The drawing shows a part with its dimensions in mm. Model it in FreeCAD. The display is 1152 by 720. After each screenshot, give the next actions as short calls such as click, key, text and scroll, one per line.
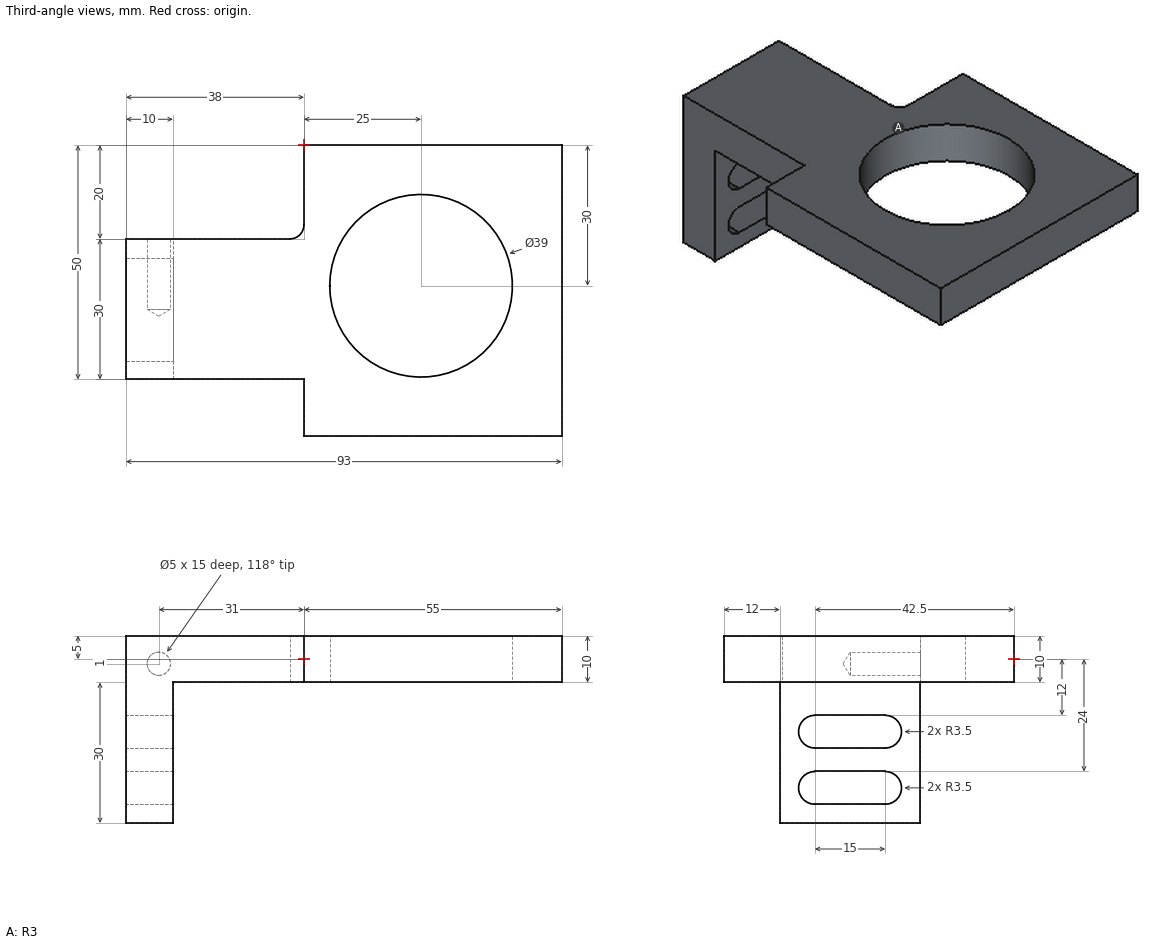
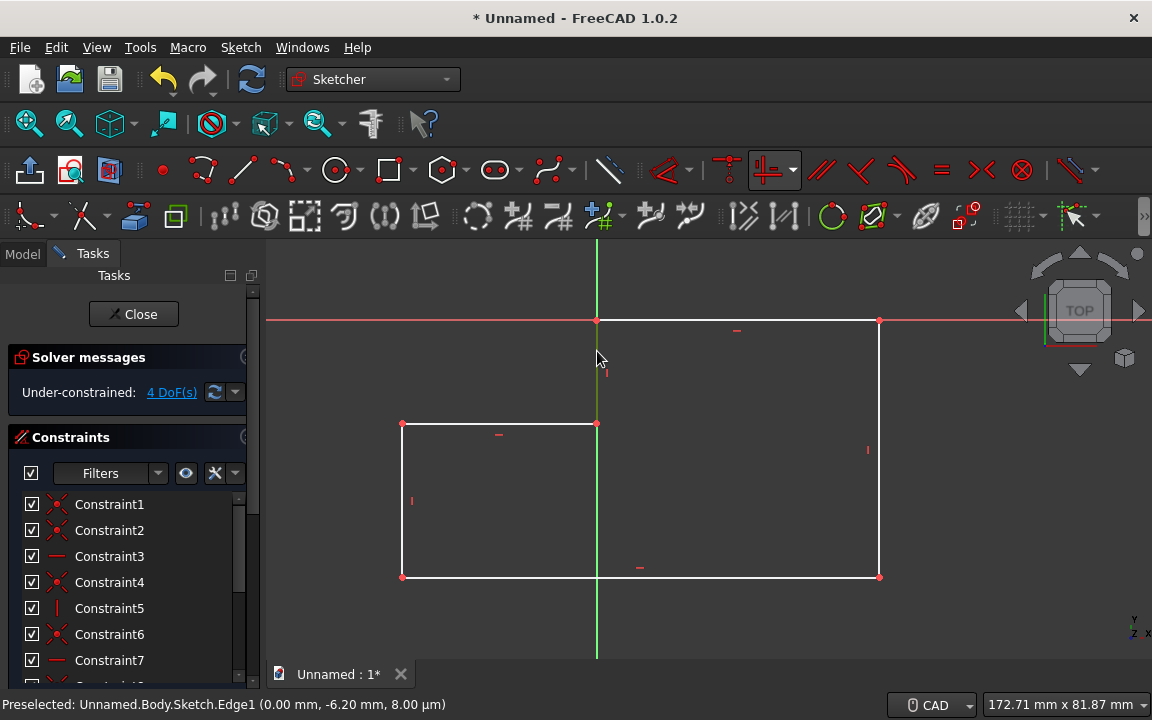
key(i)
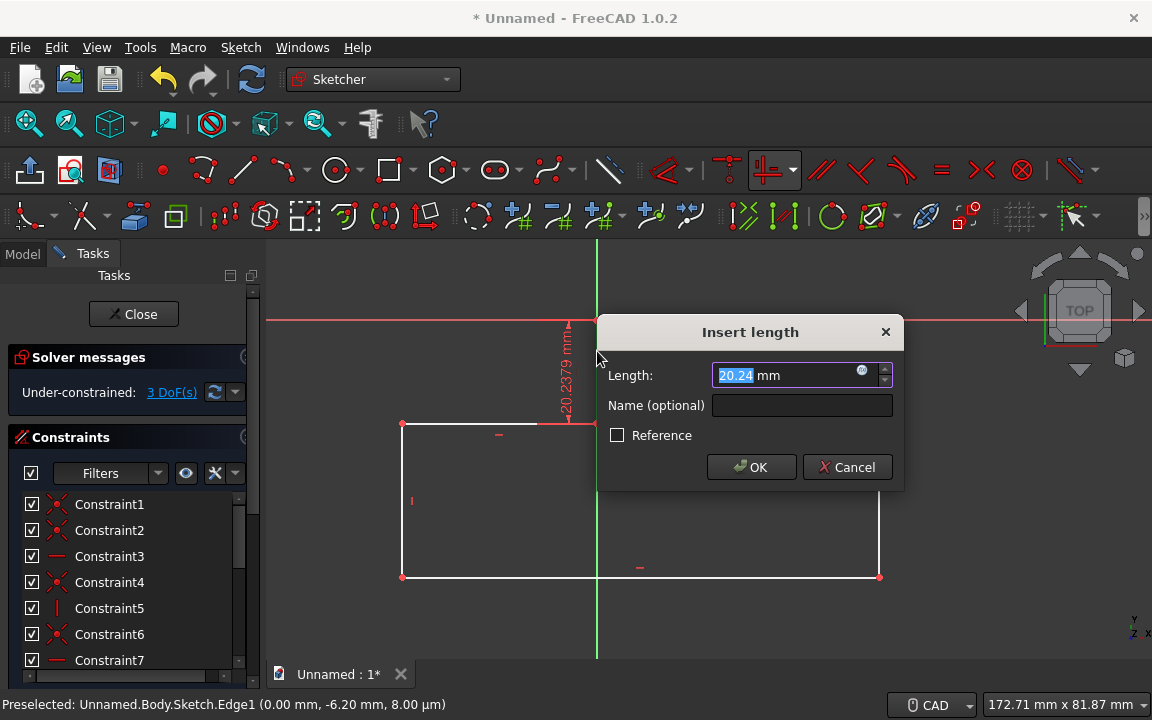
text(20)
key(Return)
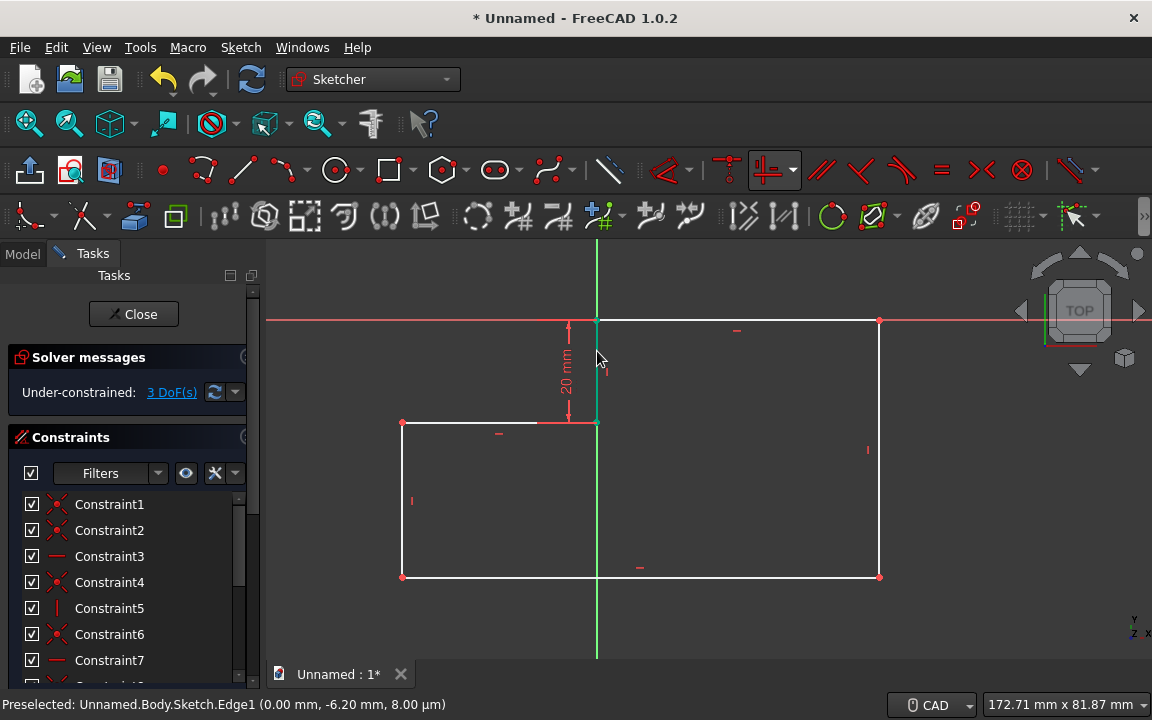
click(538, 423)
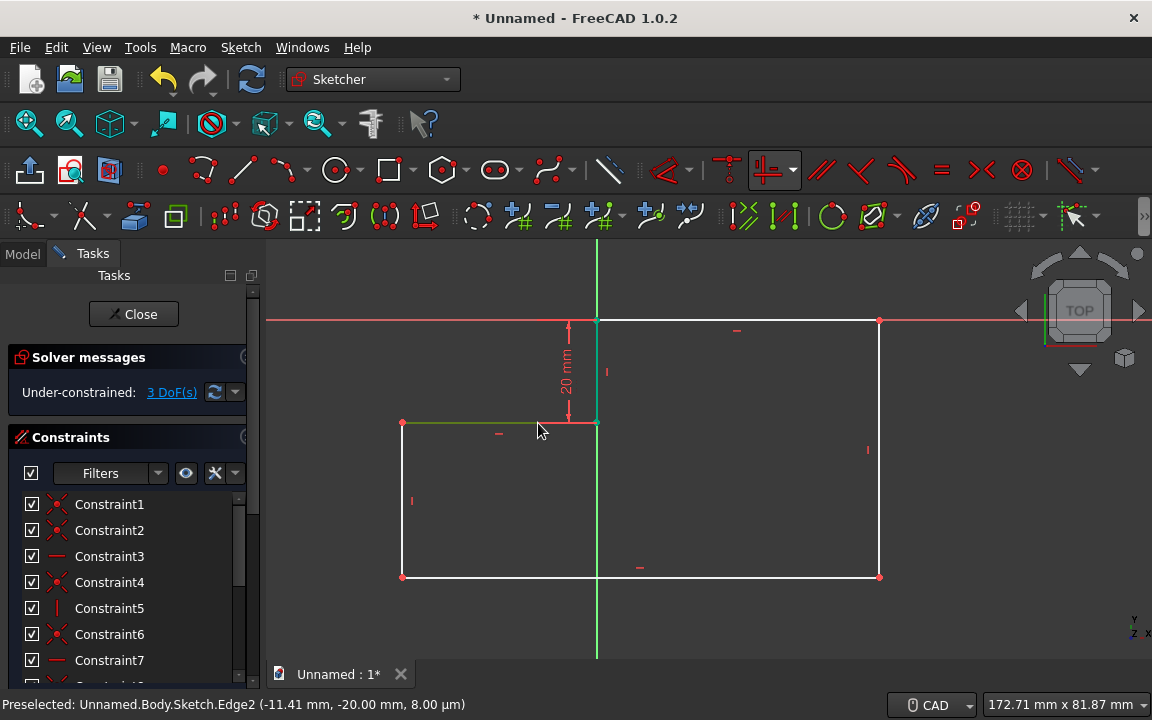
click(692, 170)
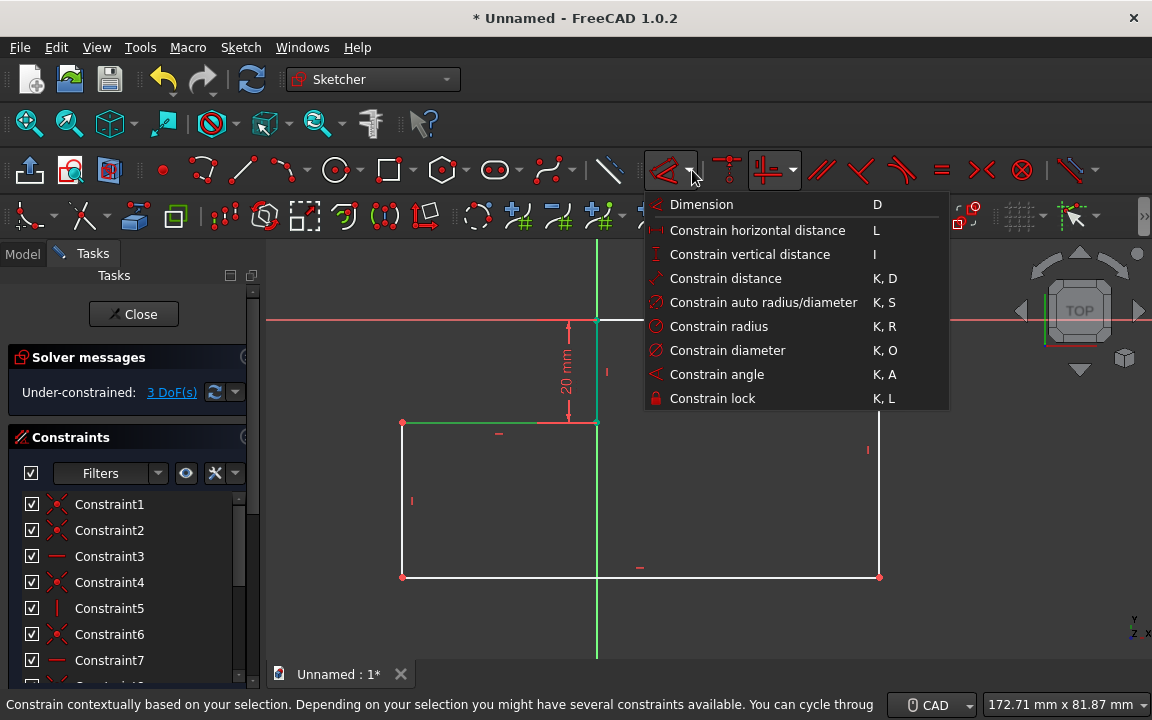
click(797, 230)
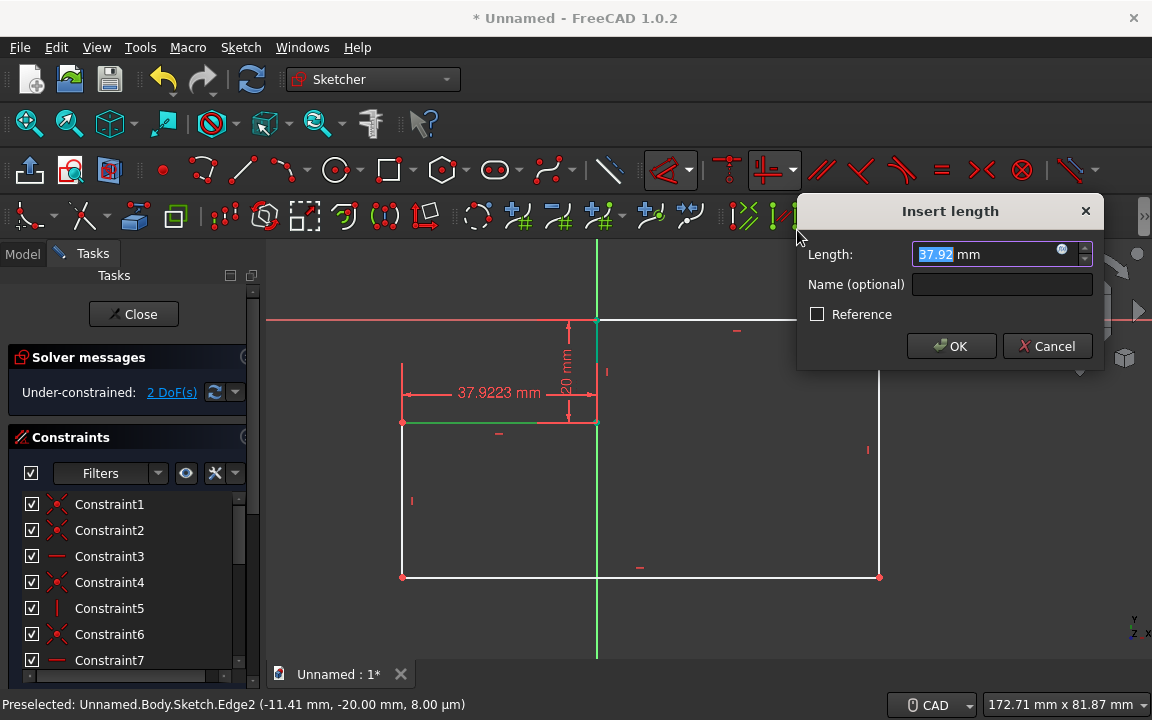
text(38)
key(Return)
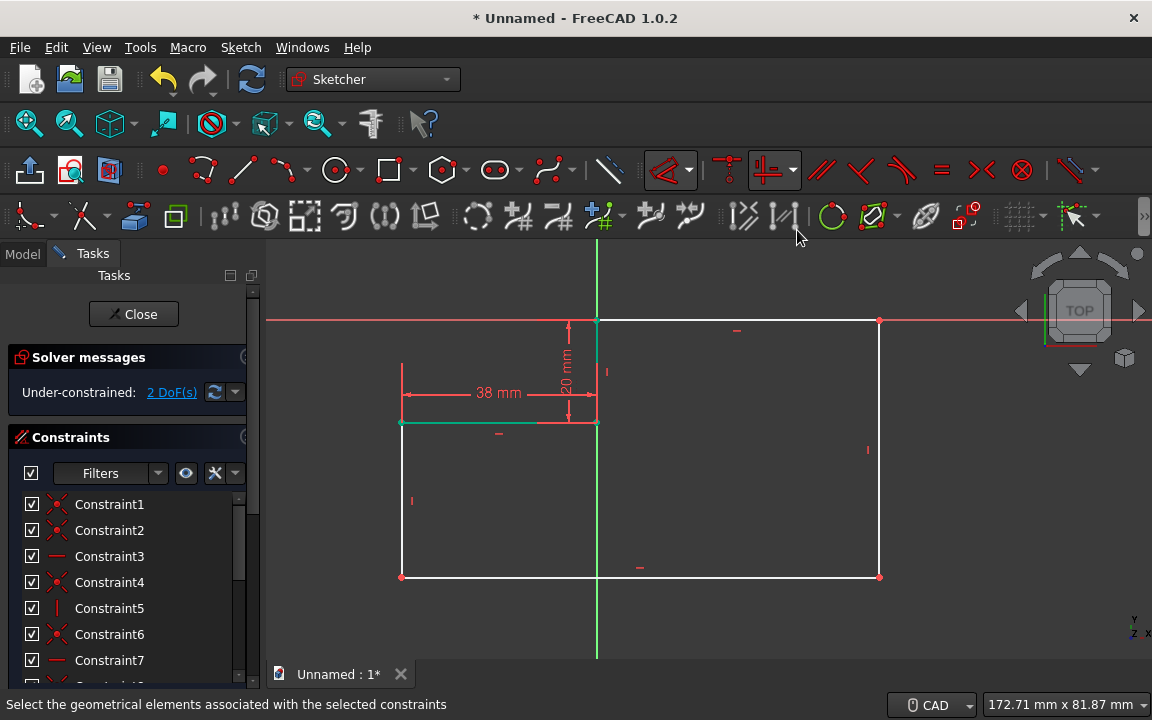
click(402, 469)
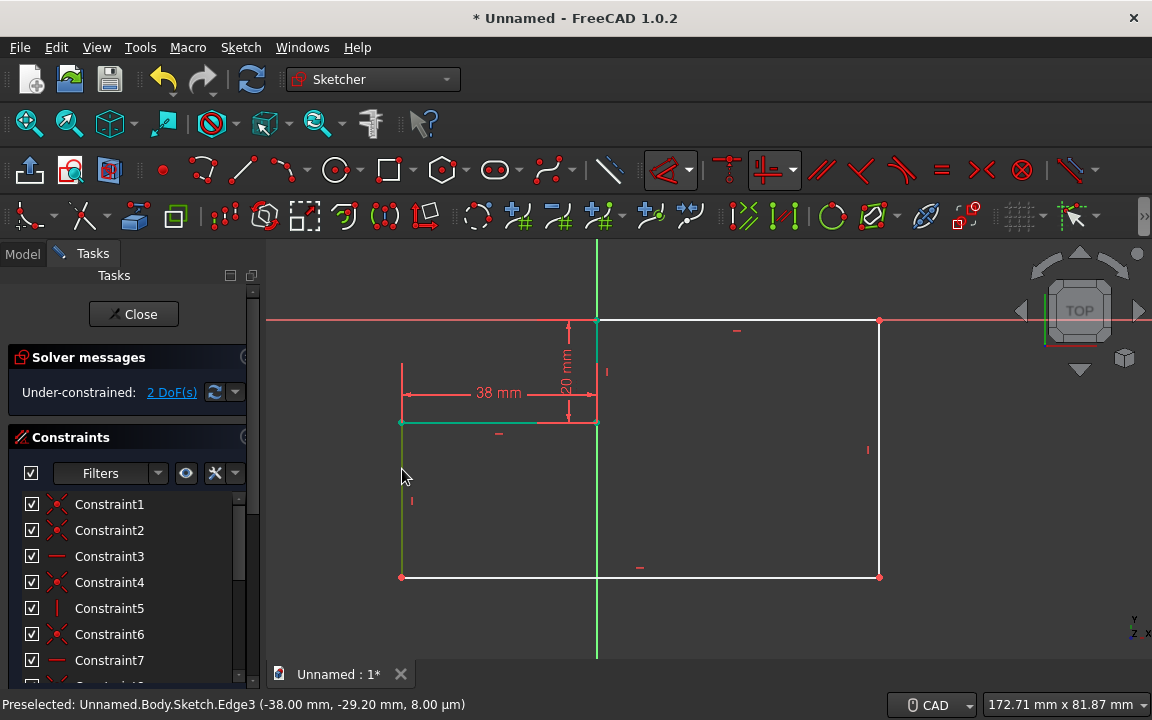
key(i)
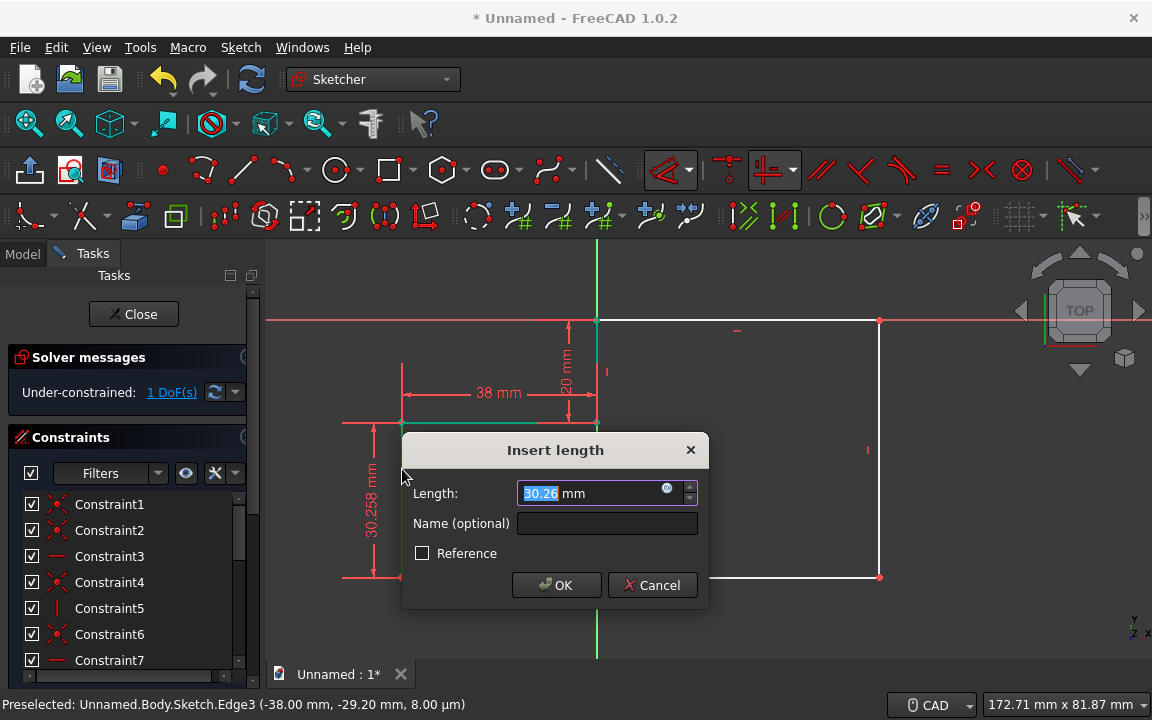
text(30)
key(Return)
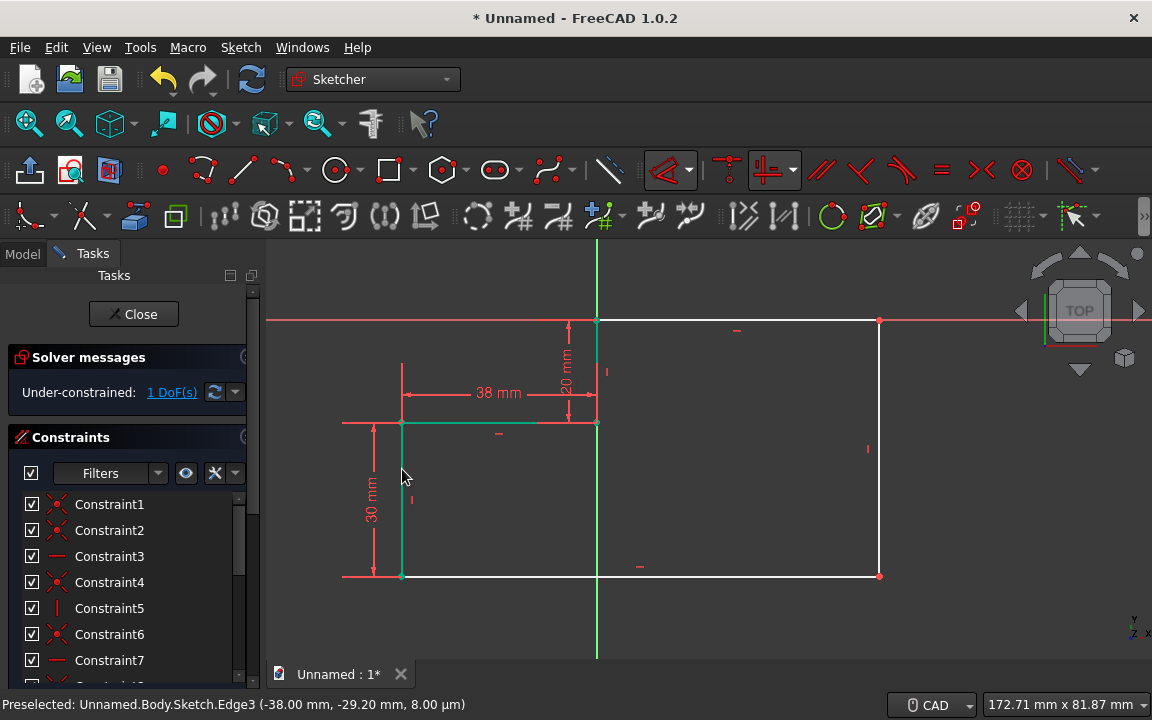
click(545, 577)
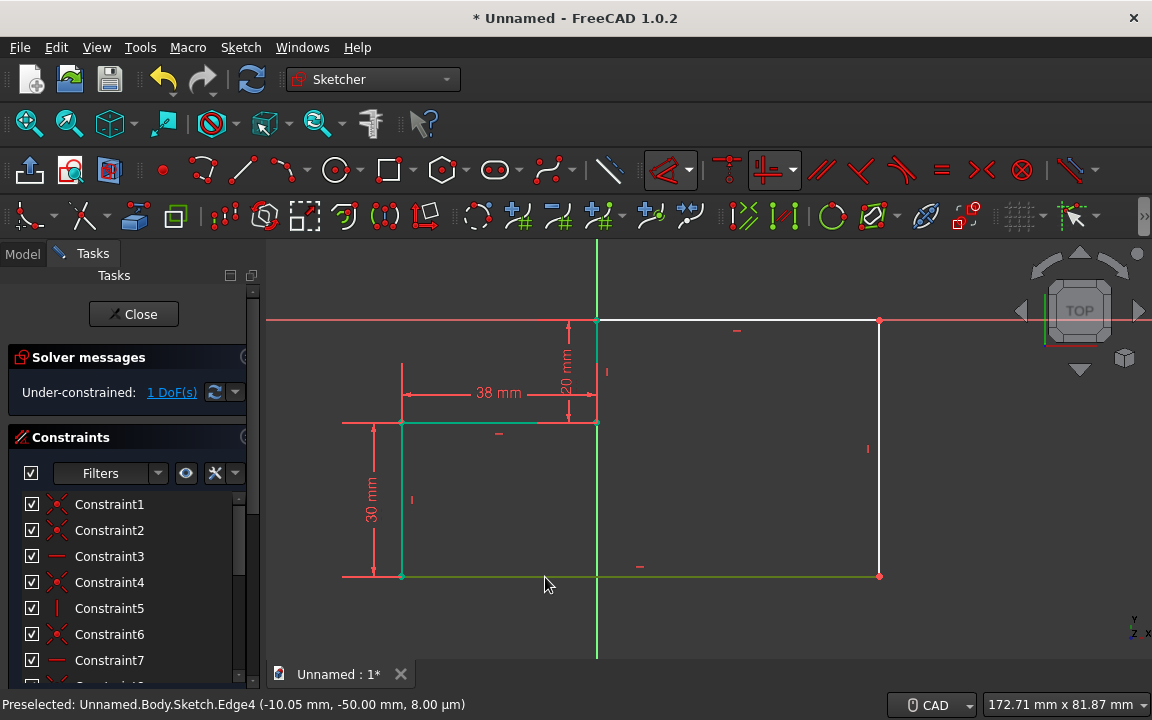
key(l)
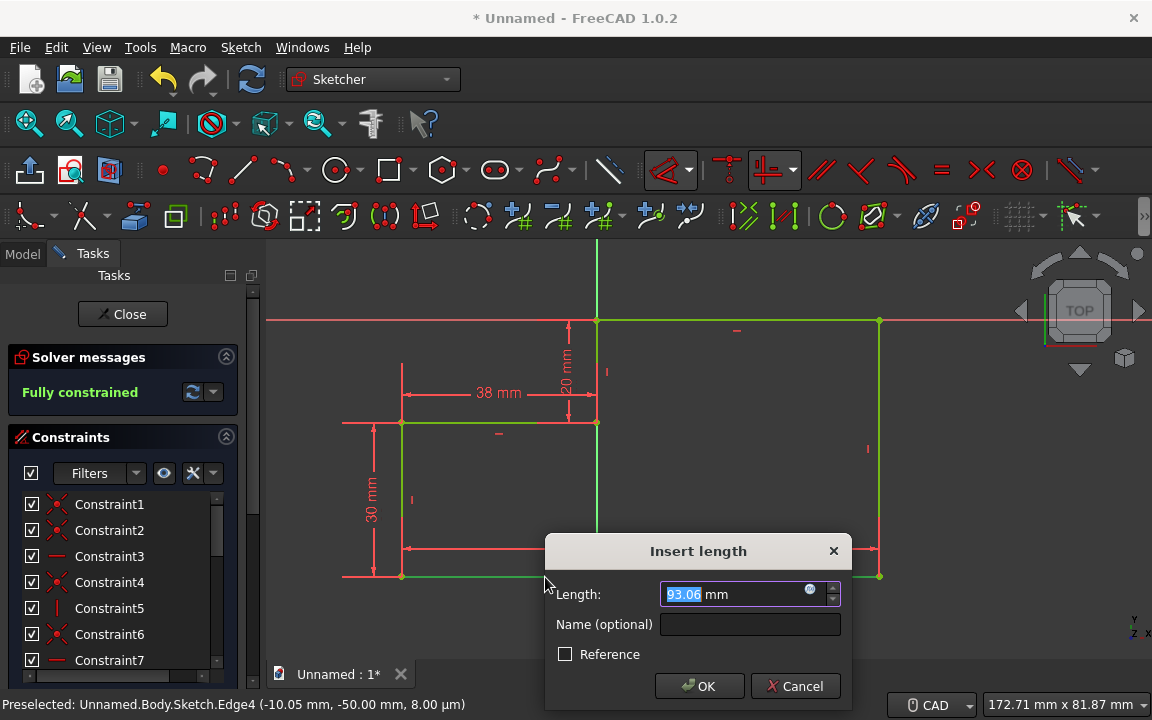
text(93)
key(Return)